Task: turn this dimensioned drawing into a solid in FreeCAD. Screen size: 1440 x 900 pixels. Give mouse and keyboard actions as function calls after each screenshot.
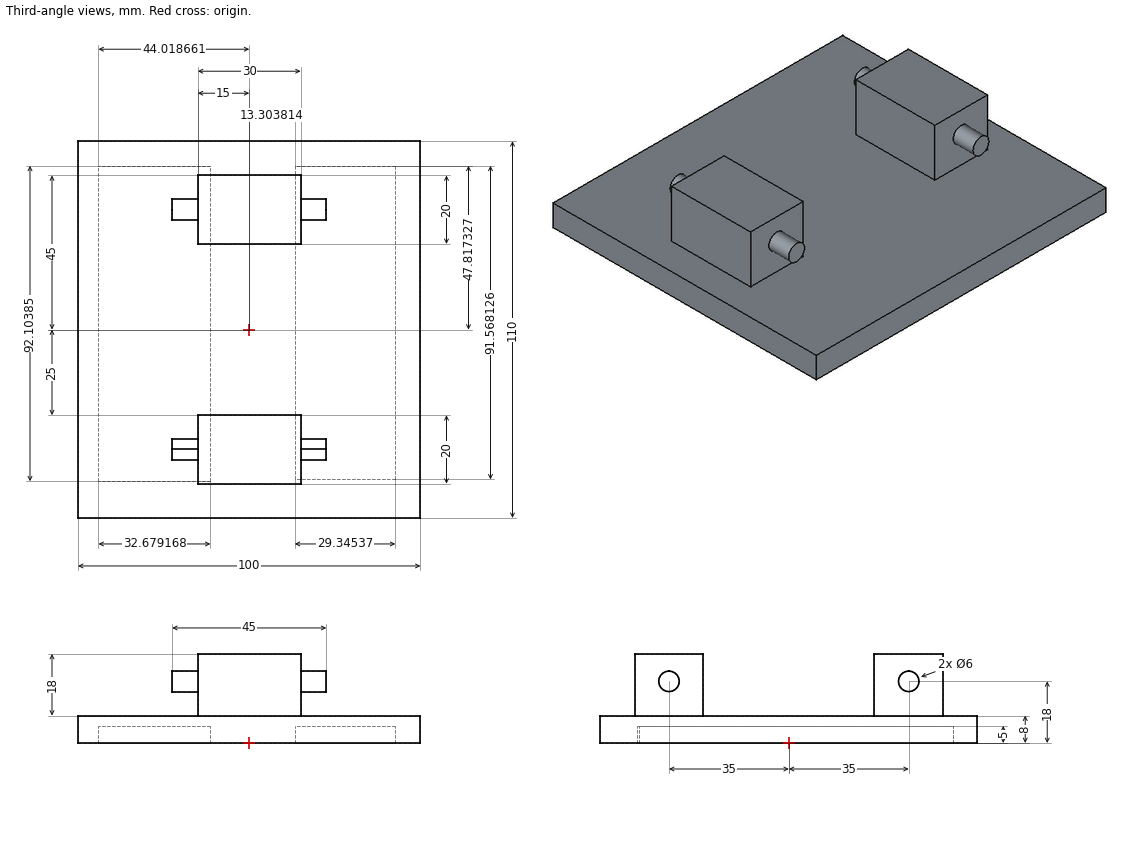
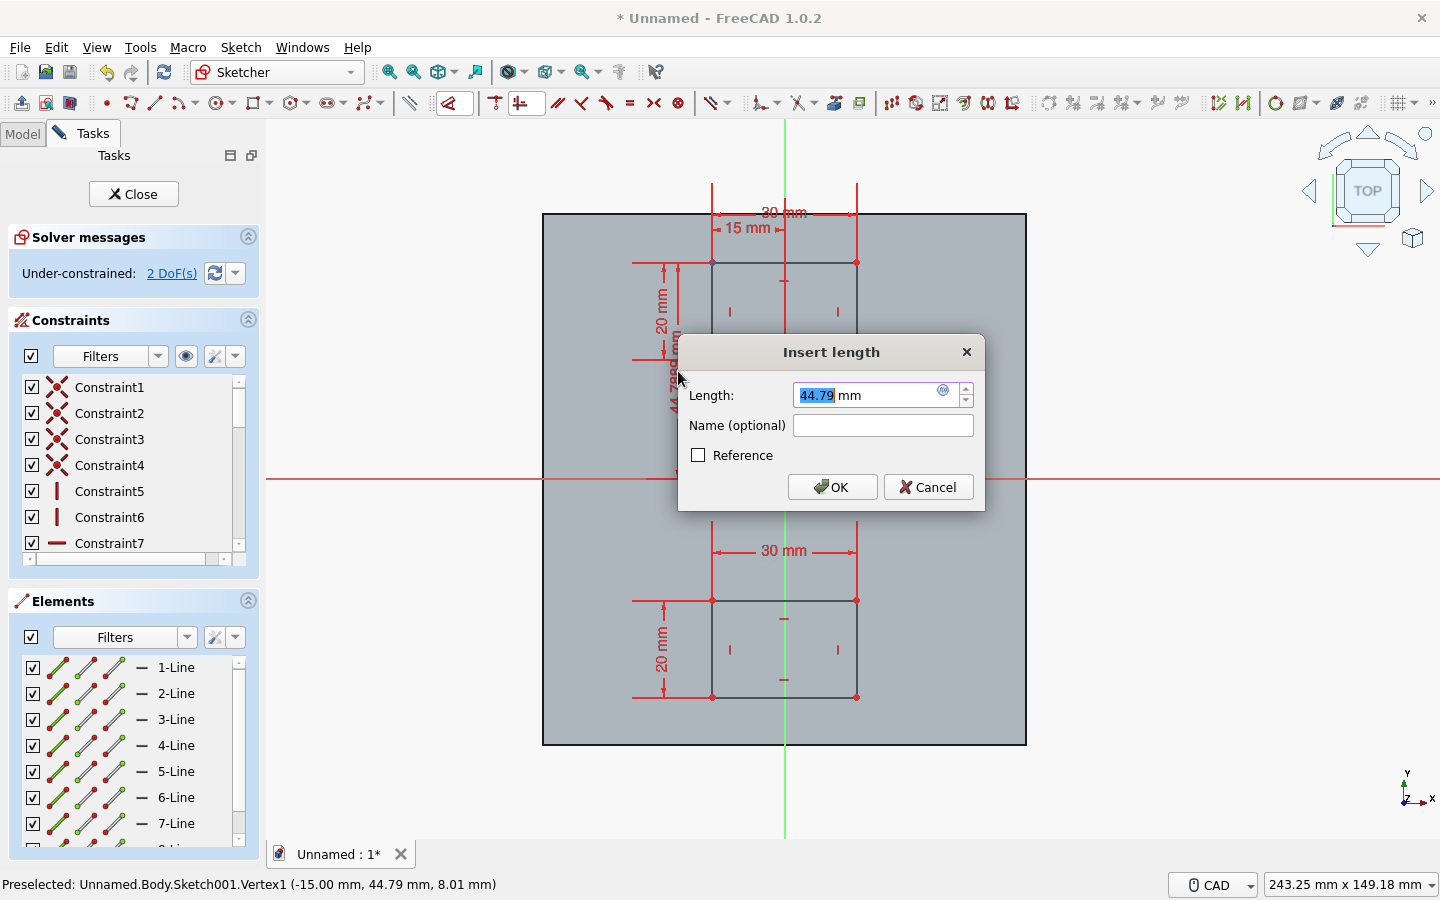
text(45)
key(Return)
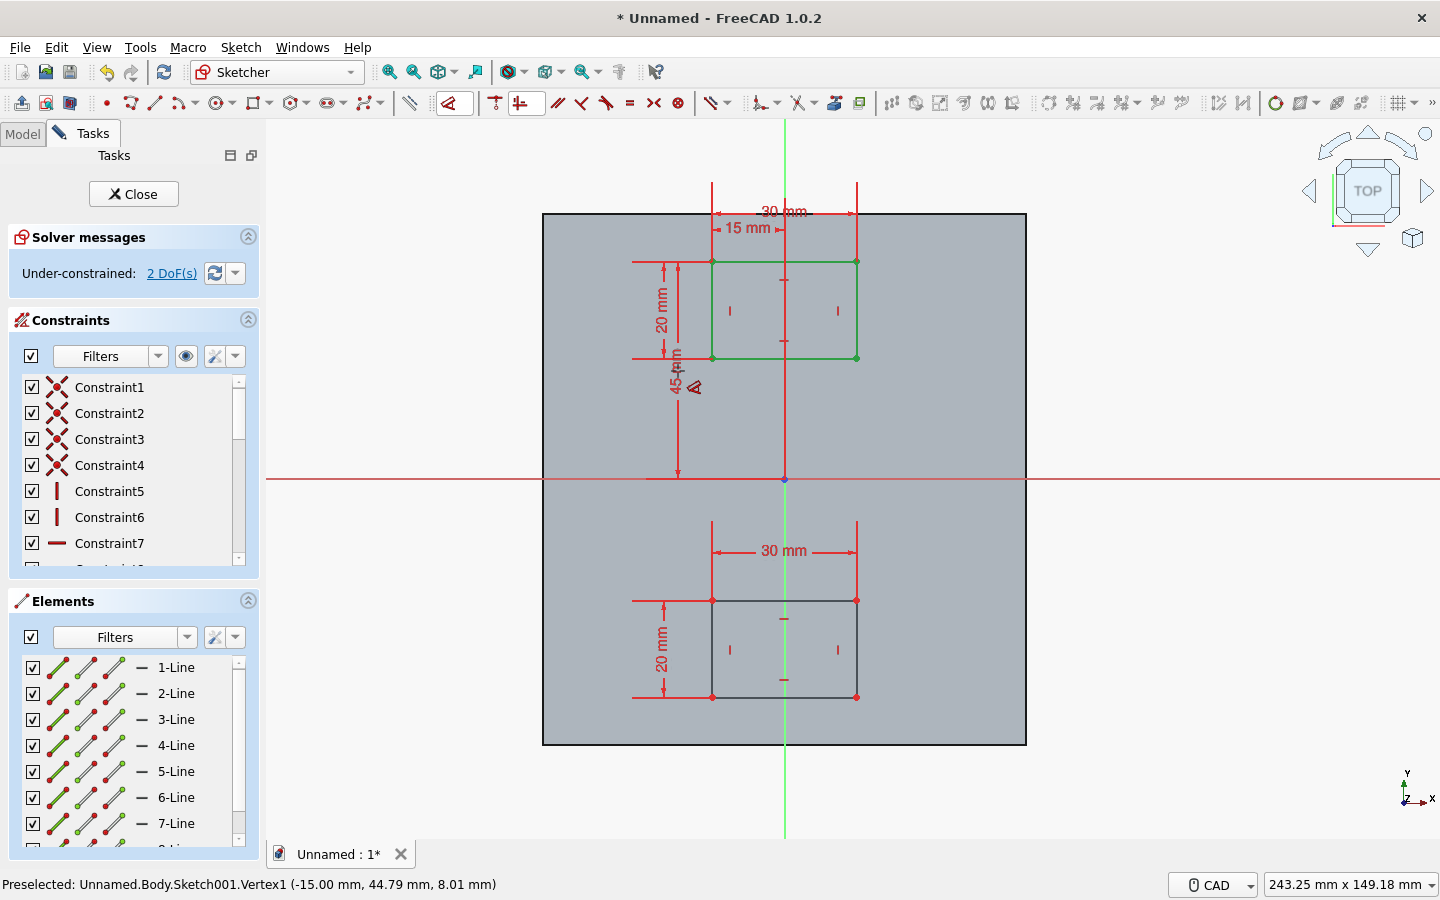
click(712, 601)
click(748, 635)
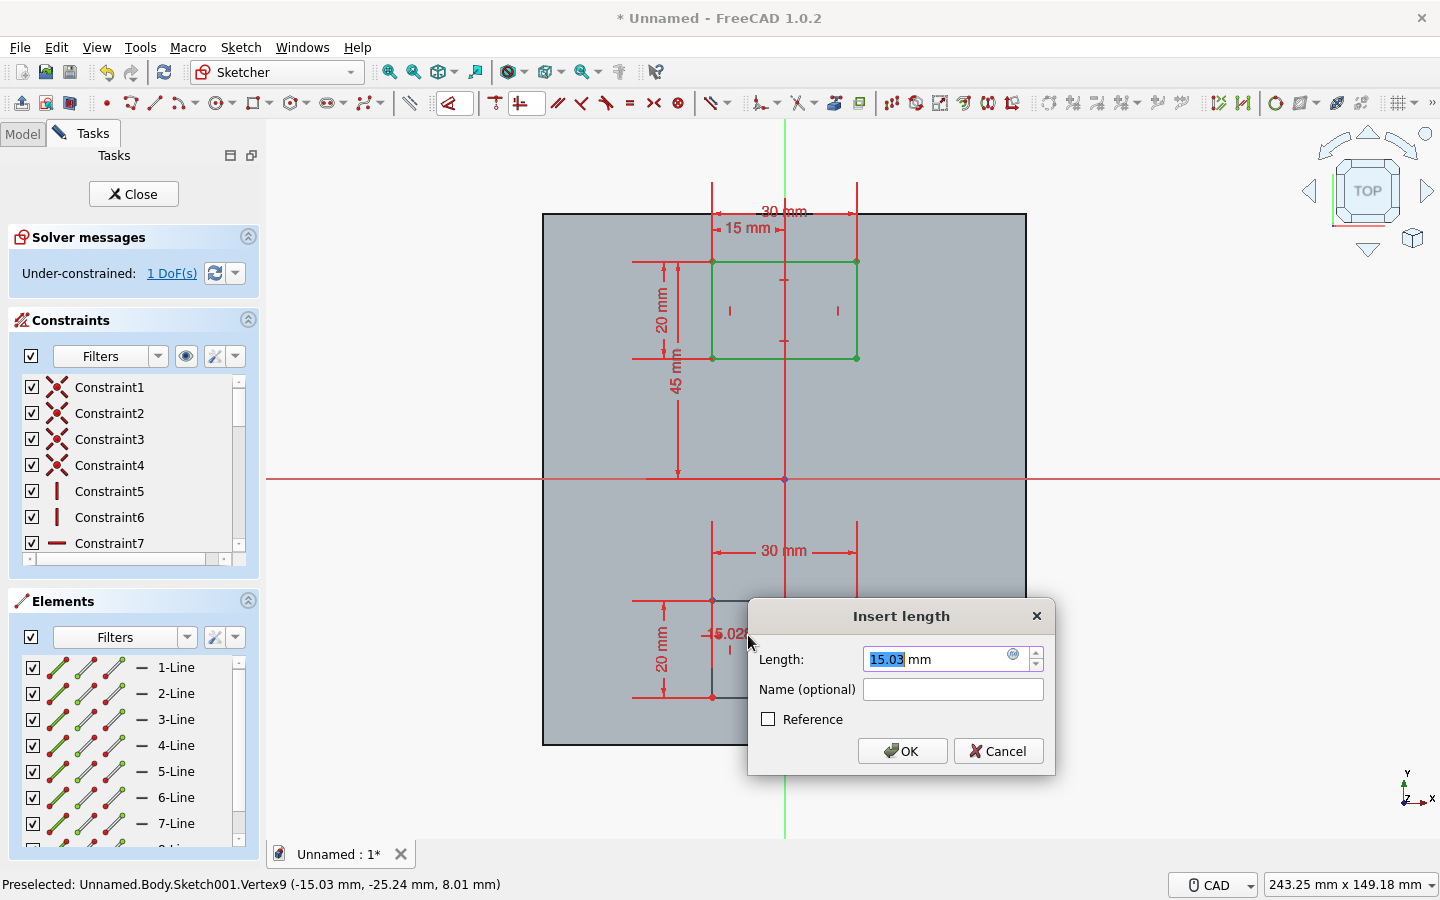
text(15)
key(Return)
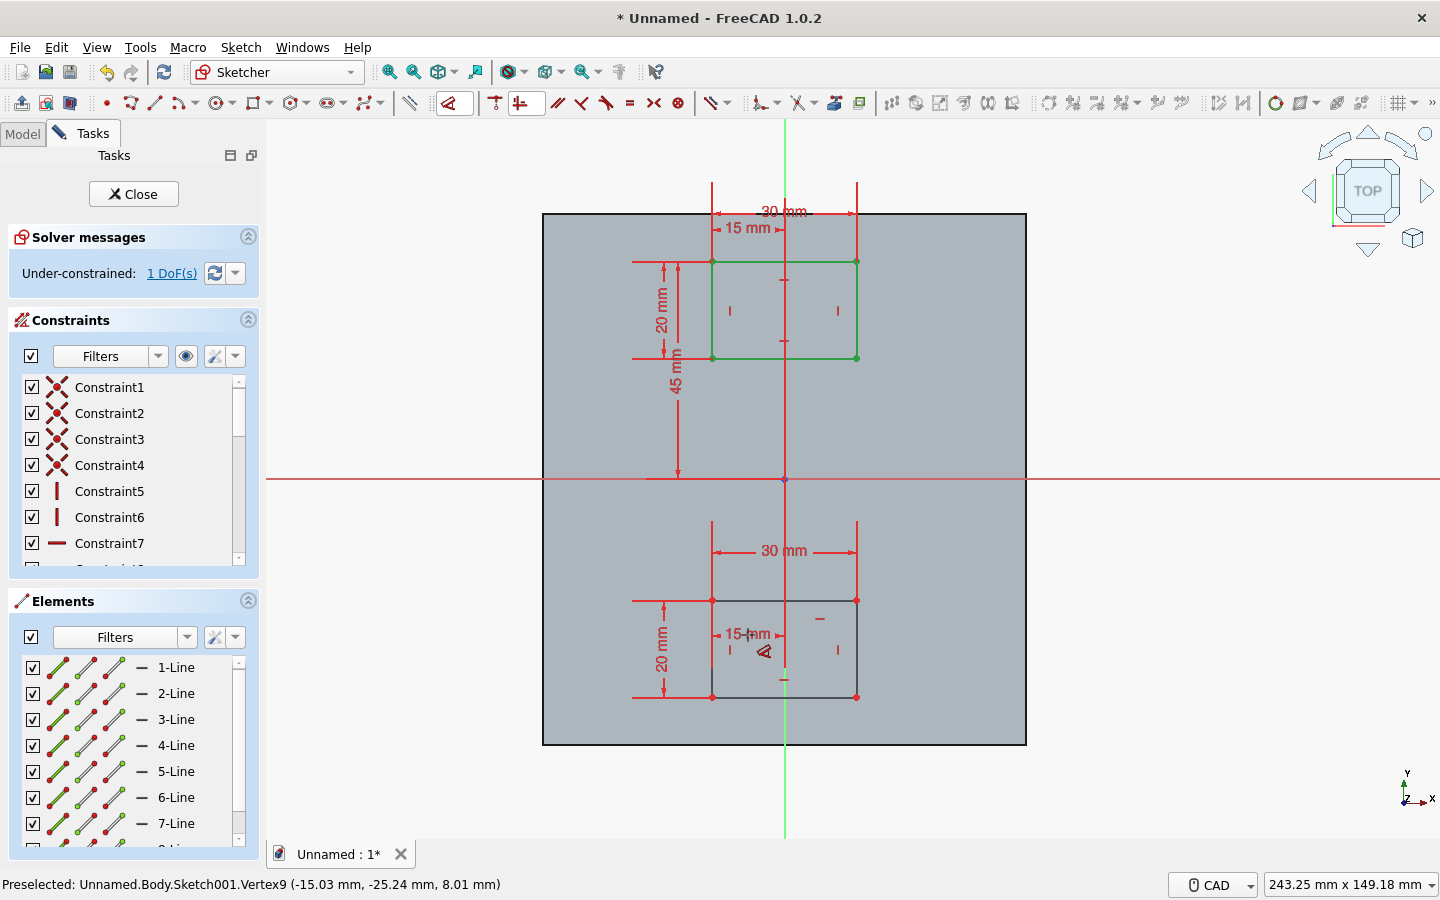
click(712, 601)
click(678, 540)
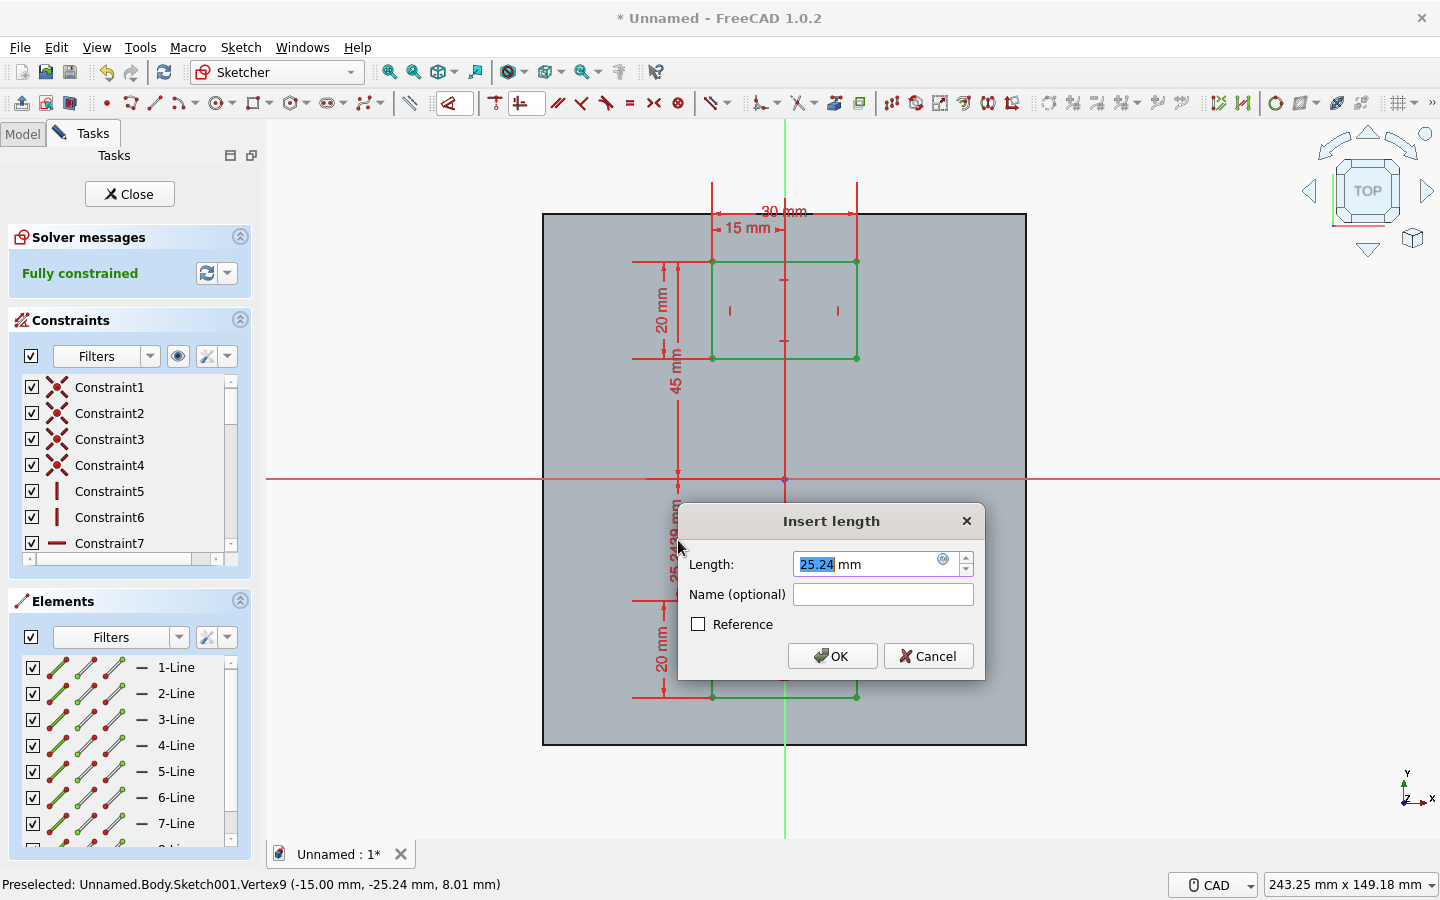
text(25)
key(Return)
key(Escape)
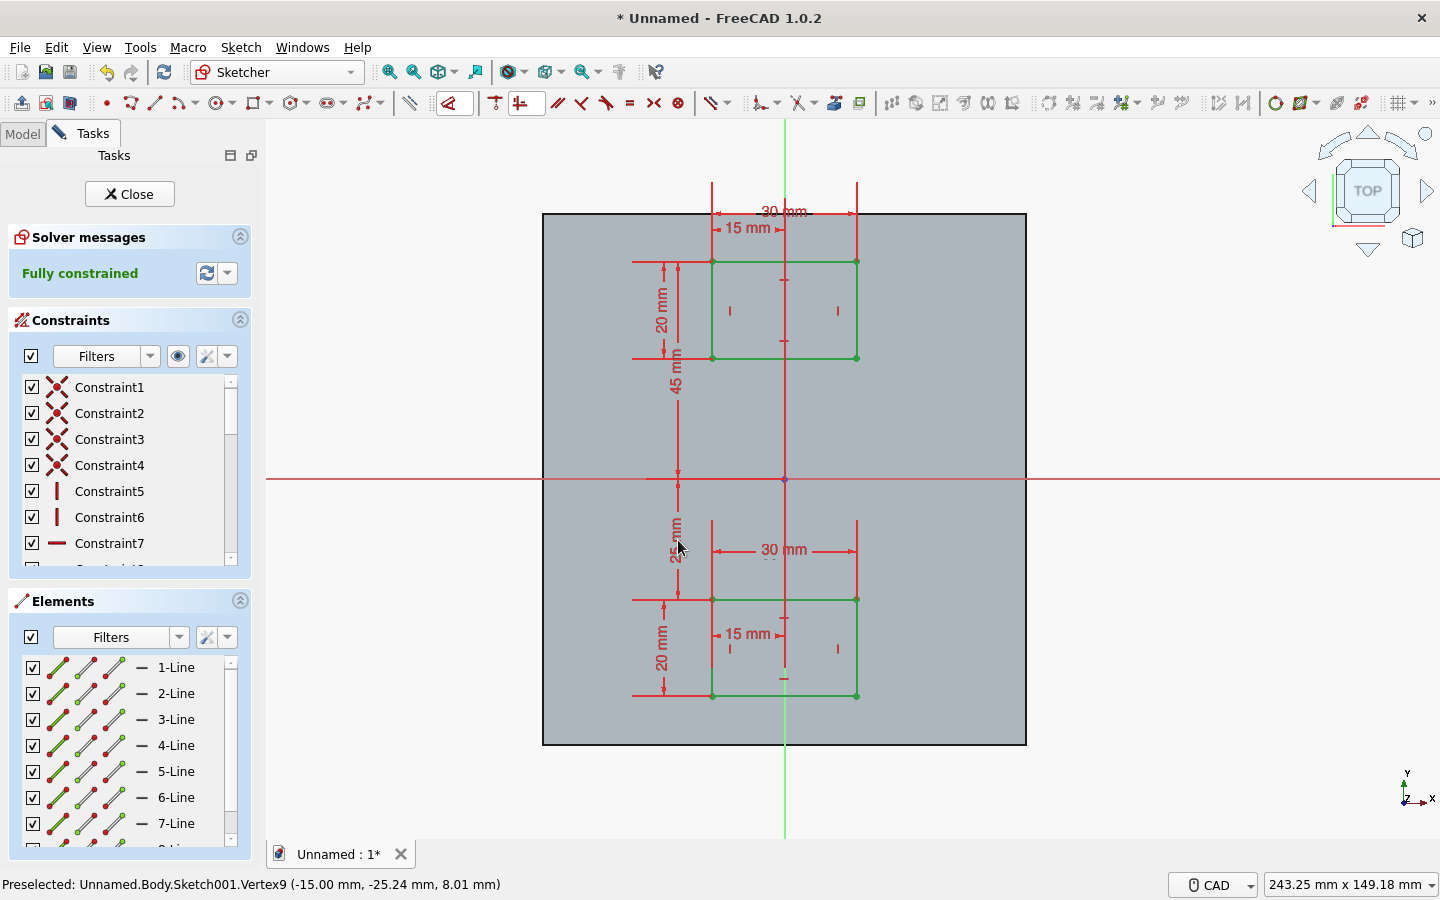
click(130, 194)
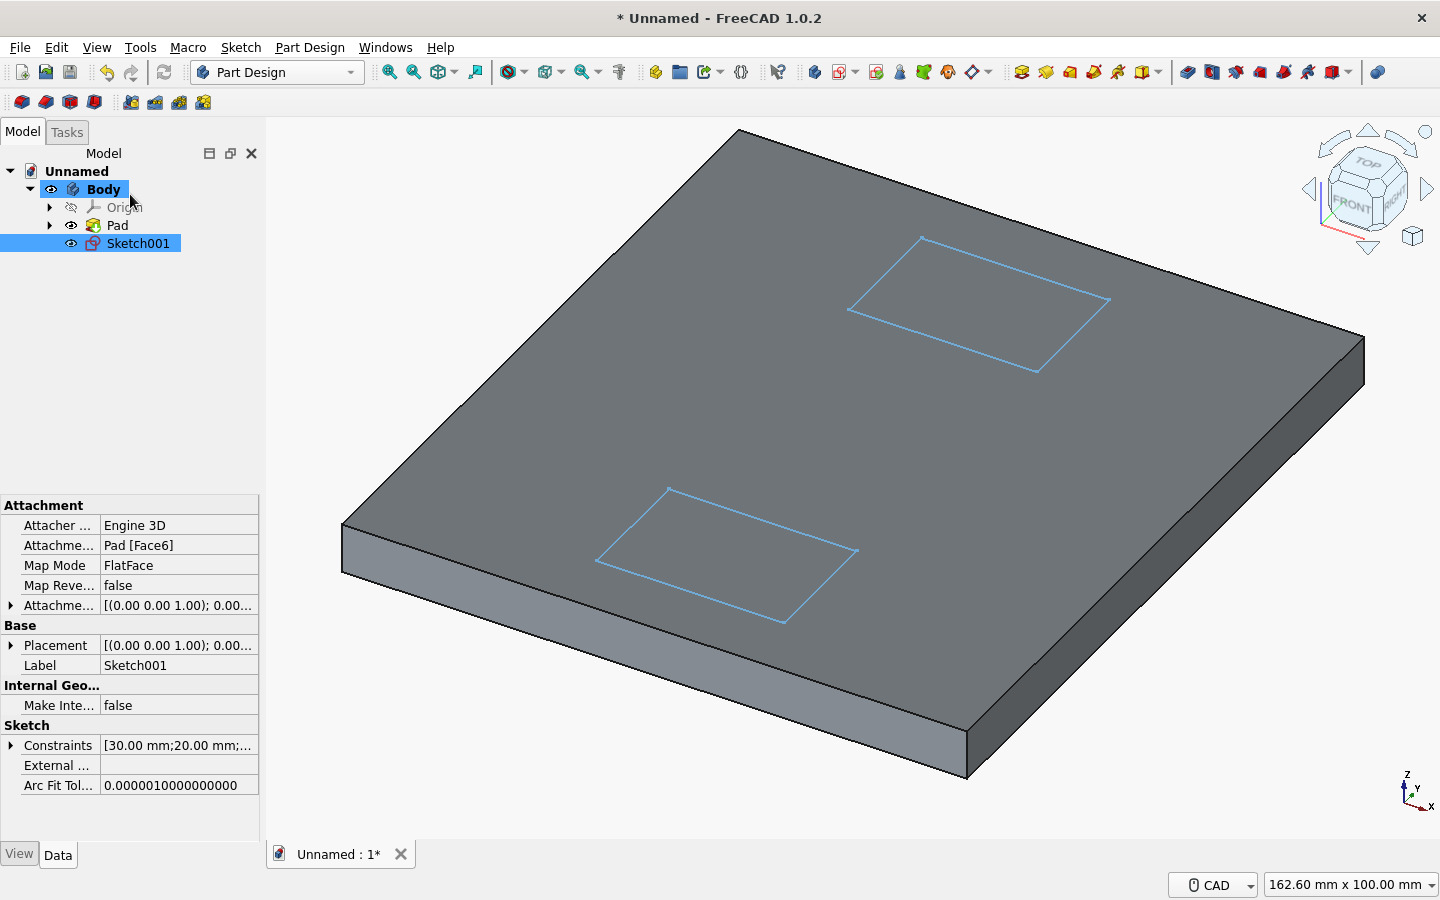
click(1022, 72)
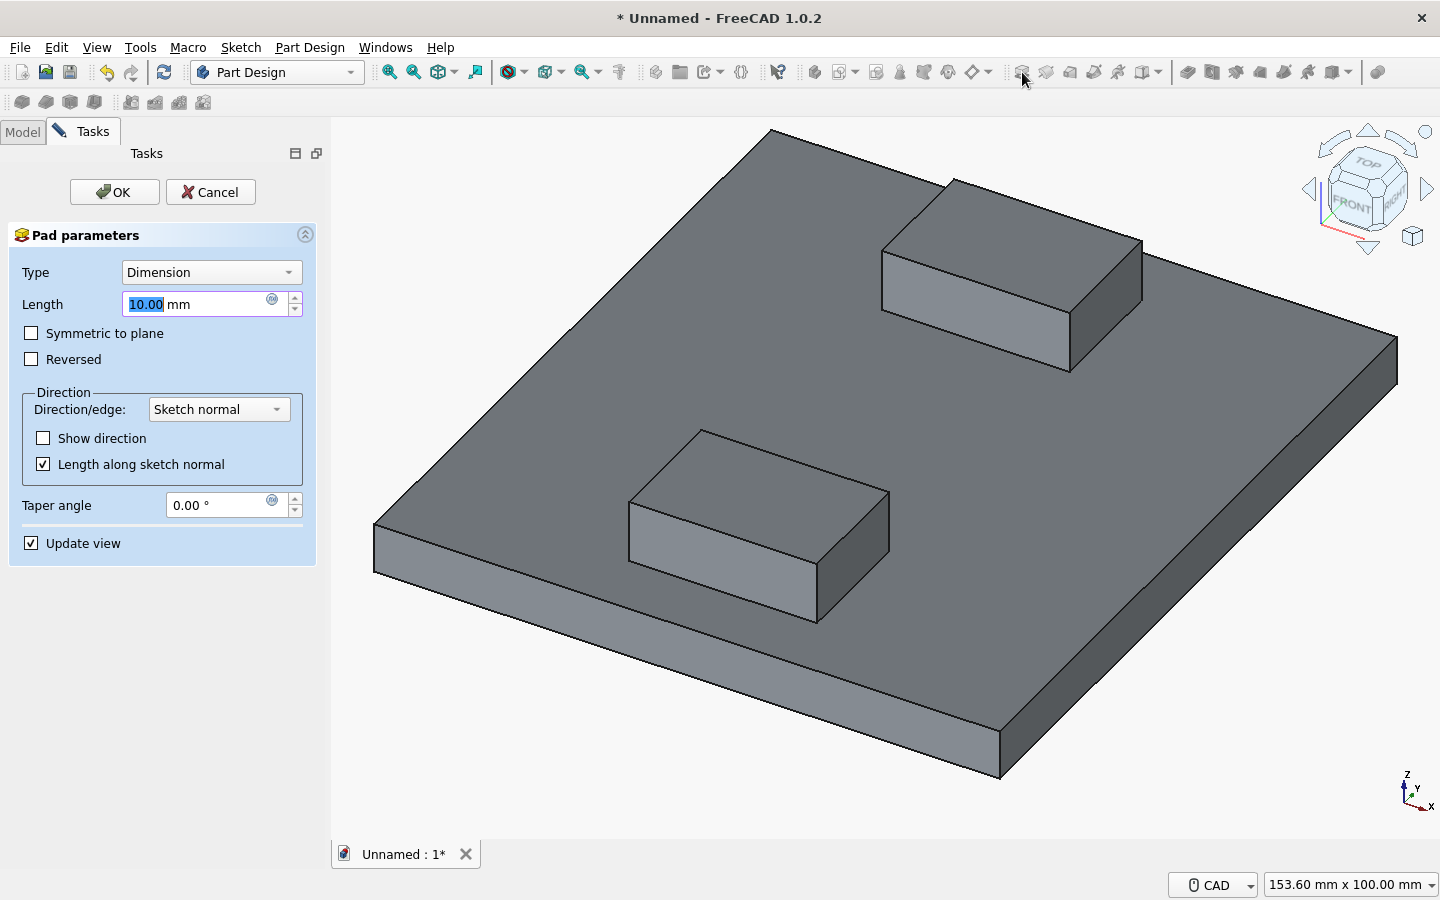
text(18)
key(Tab)